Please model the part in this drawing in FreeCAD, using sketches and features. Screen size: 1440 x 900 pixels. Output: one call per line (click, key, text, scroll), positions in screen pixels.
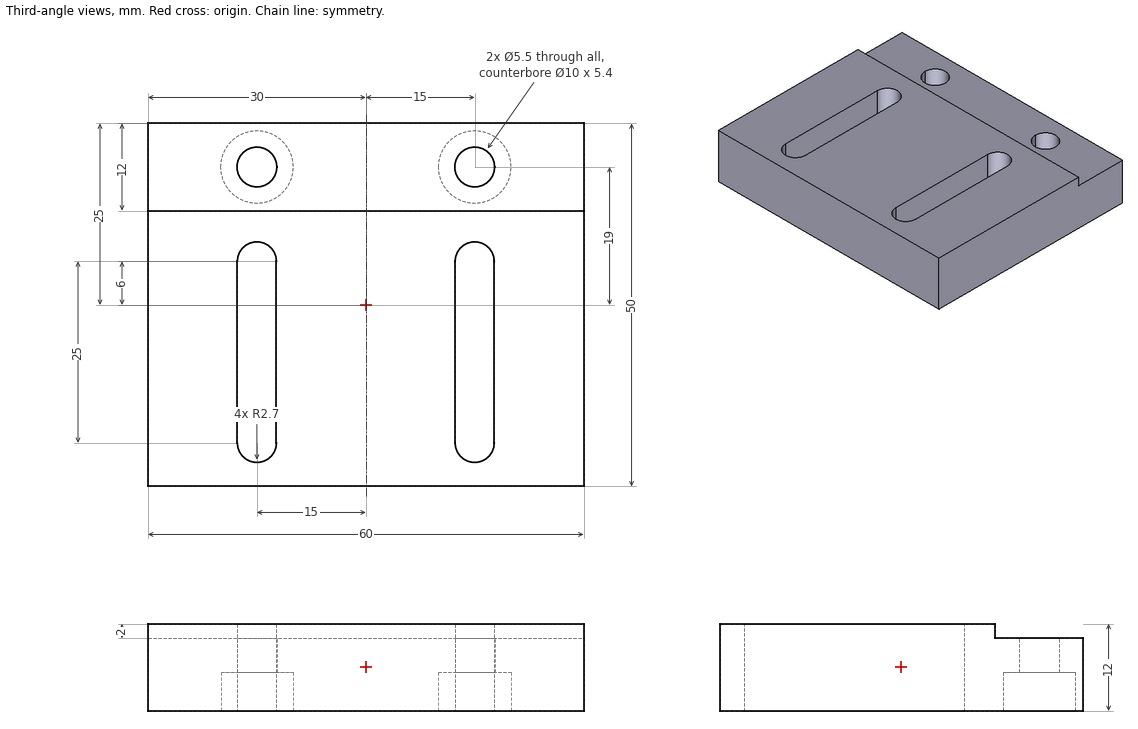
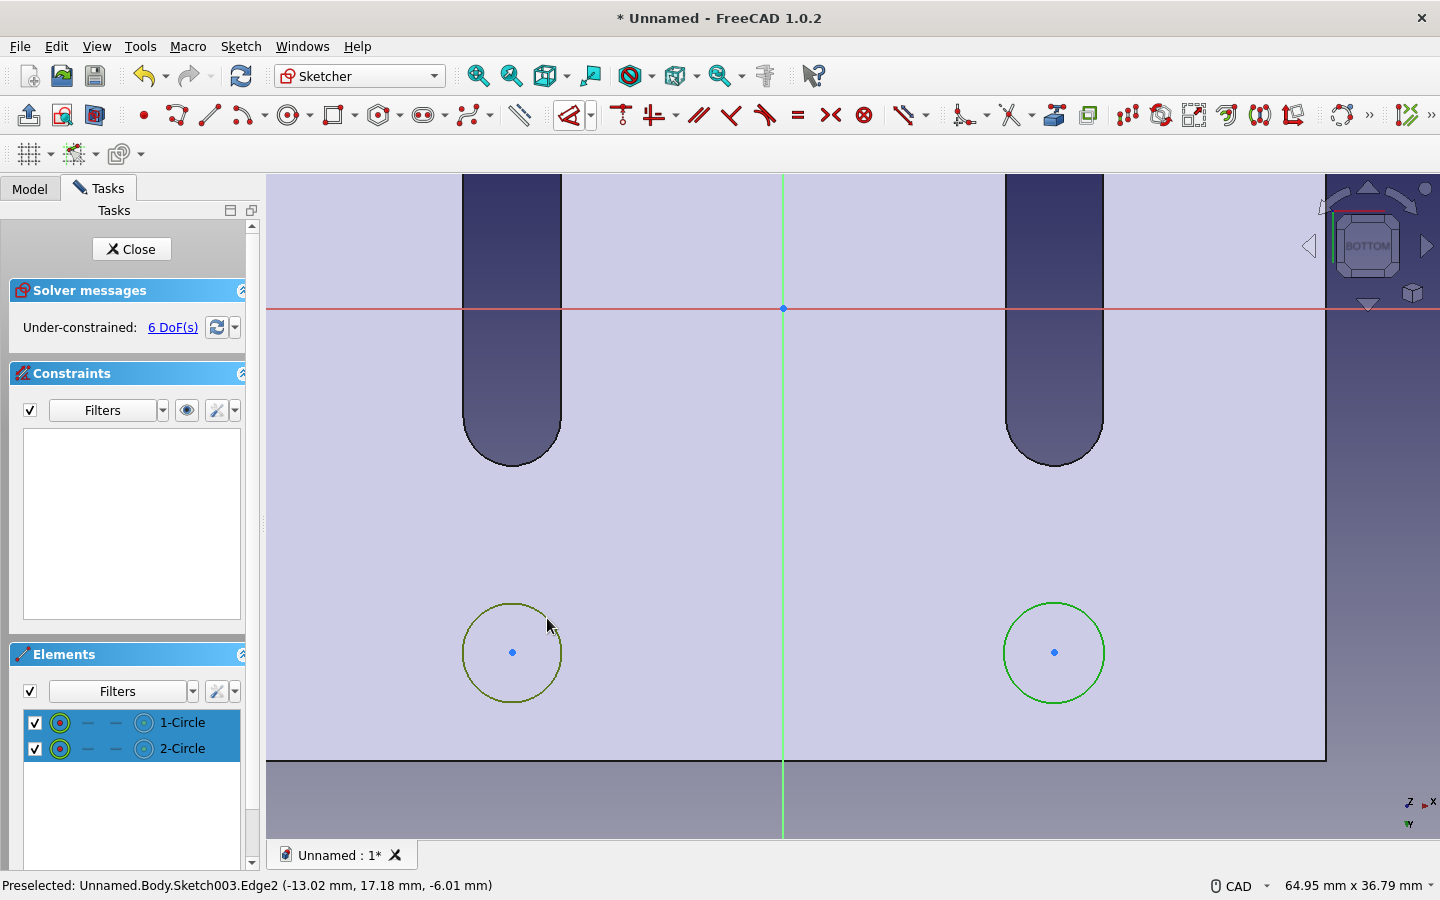
key(e)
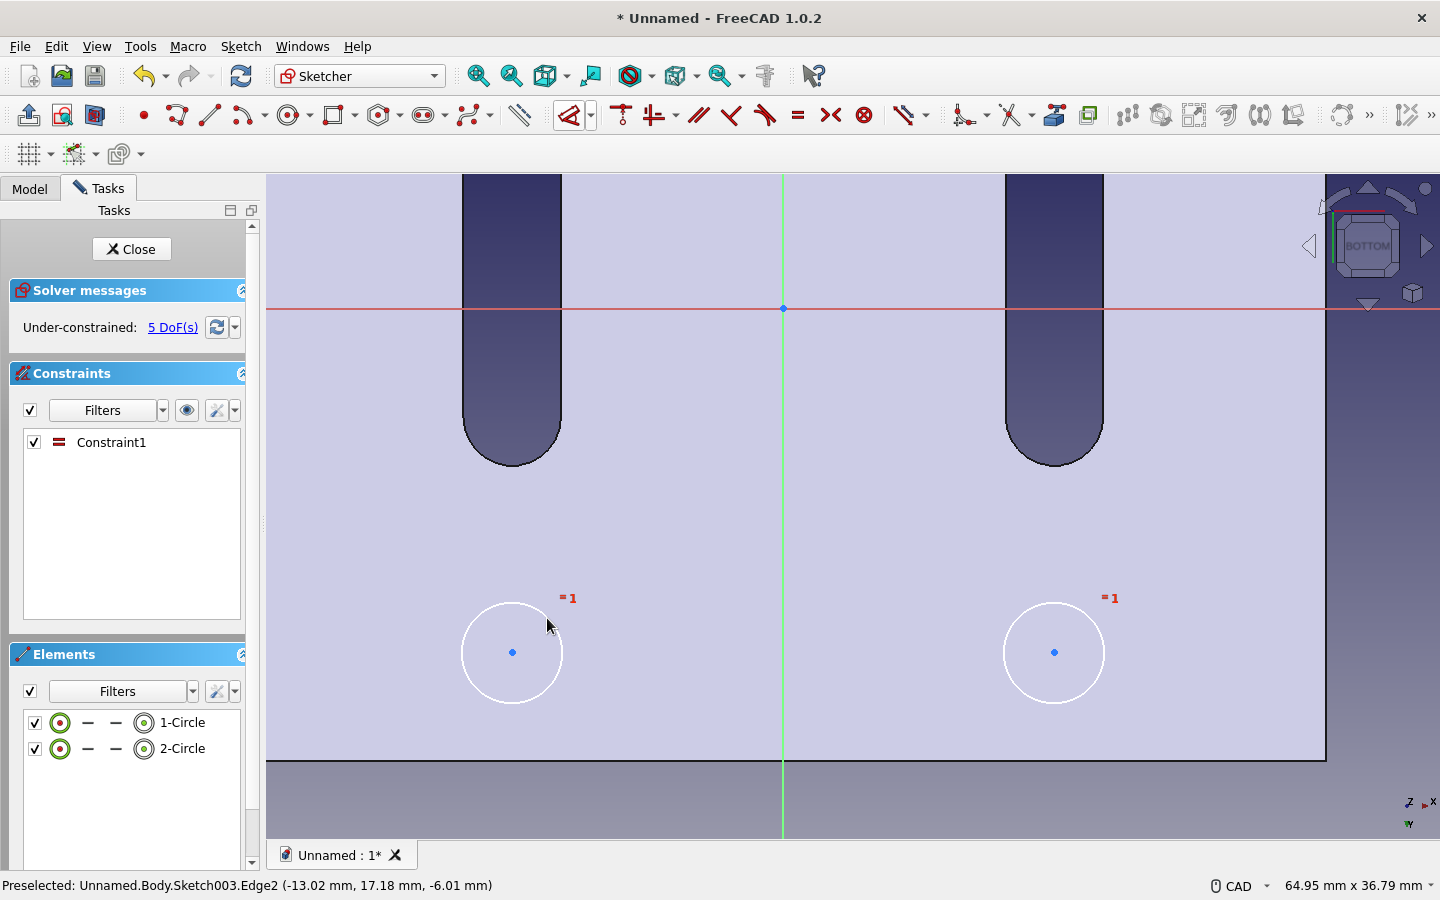
click(1054, 653)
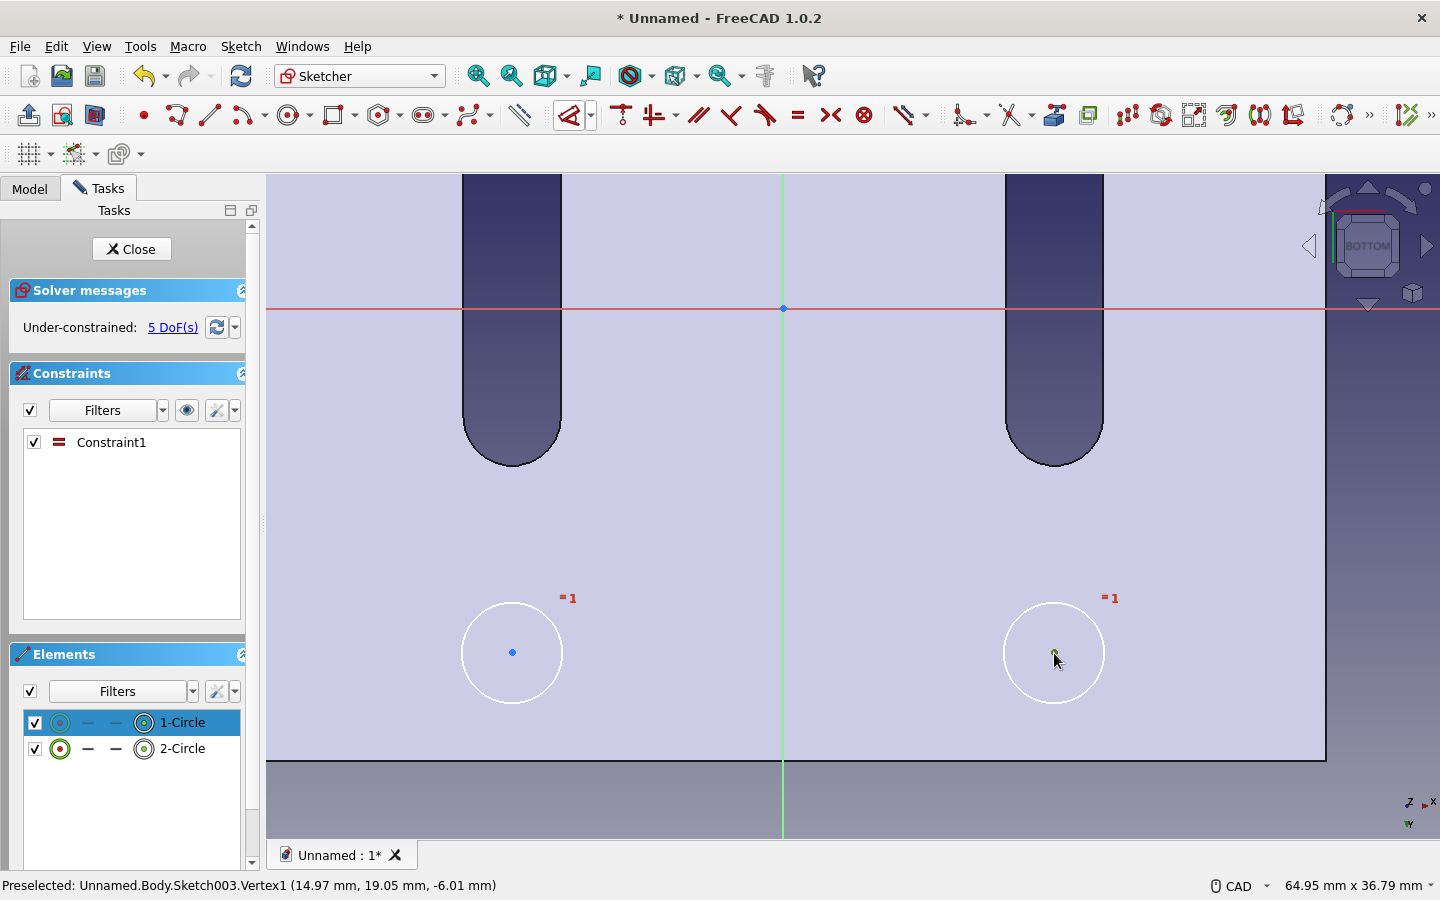
click(512, 653)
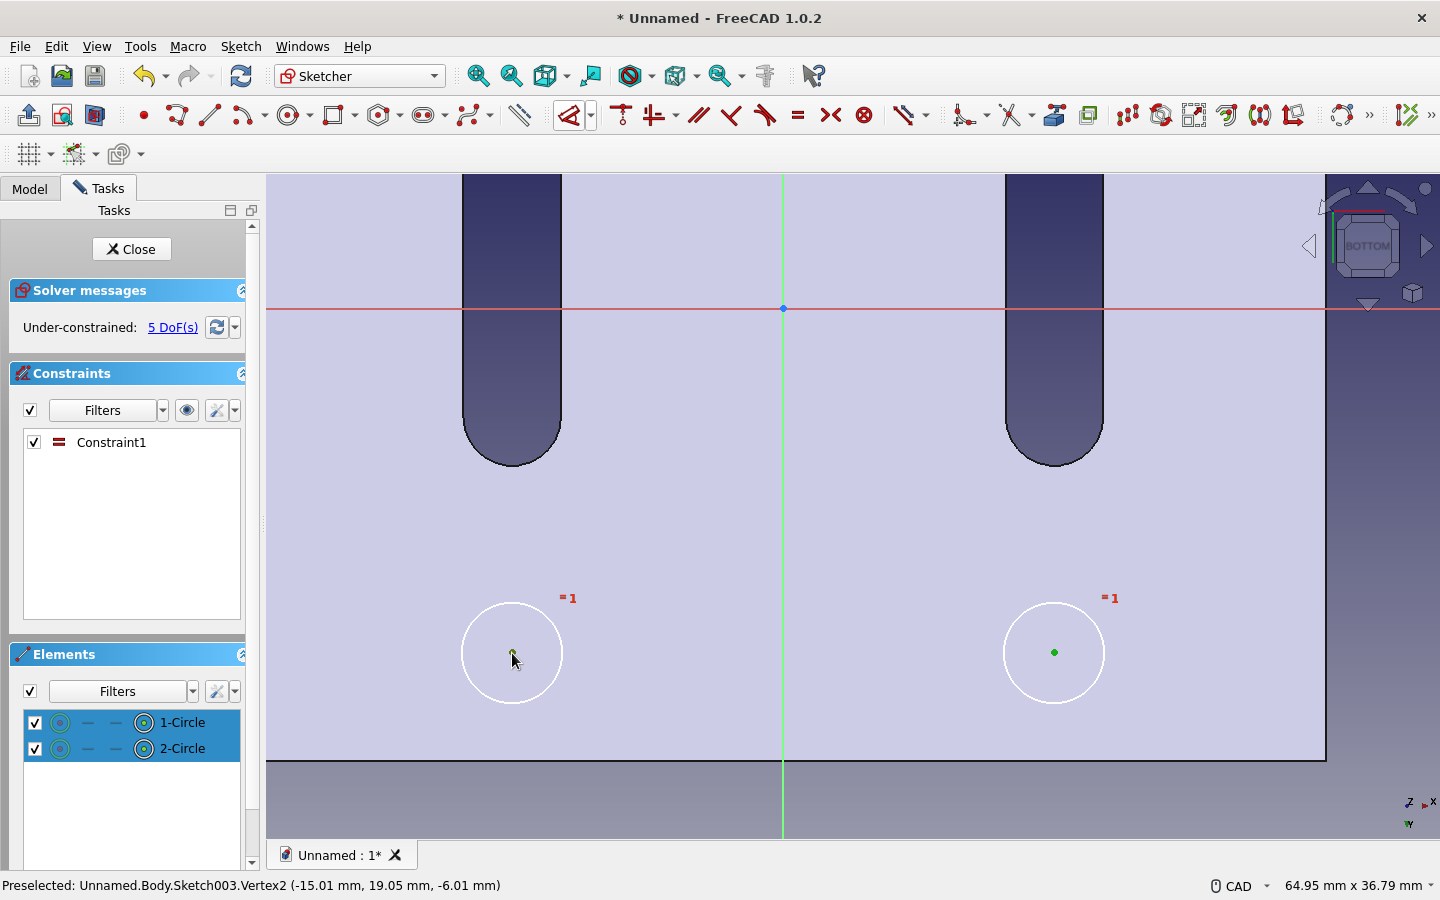
click(676, 116)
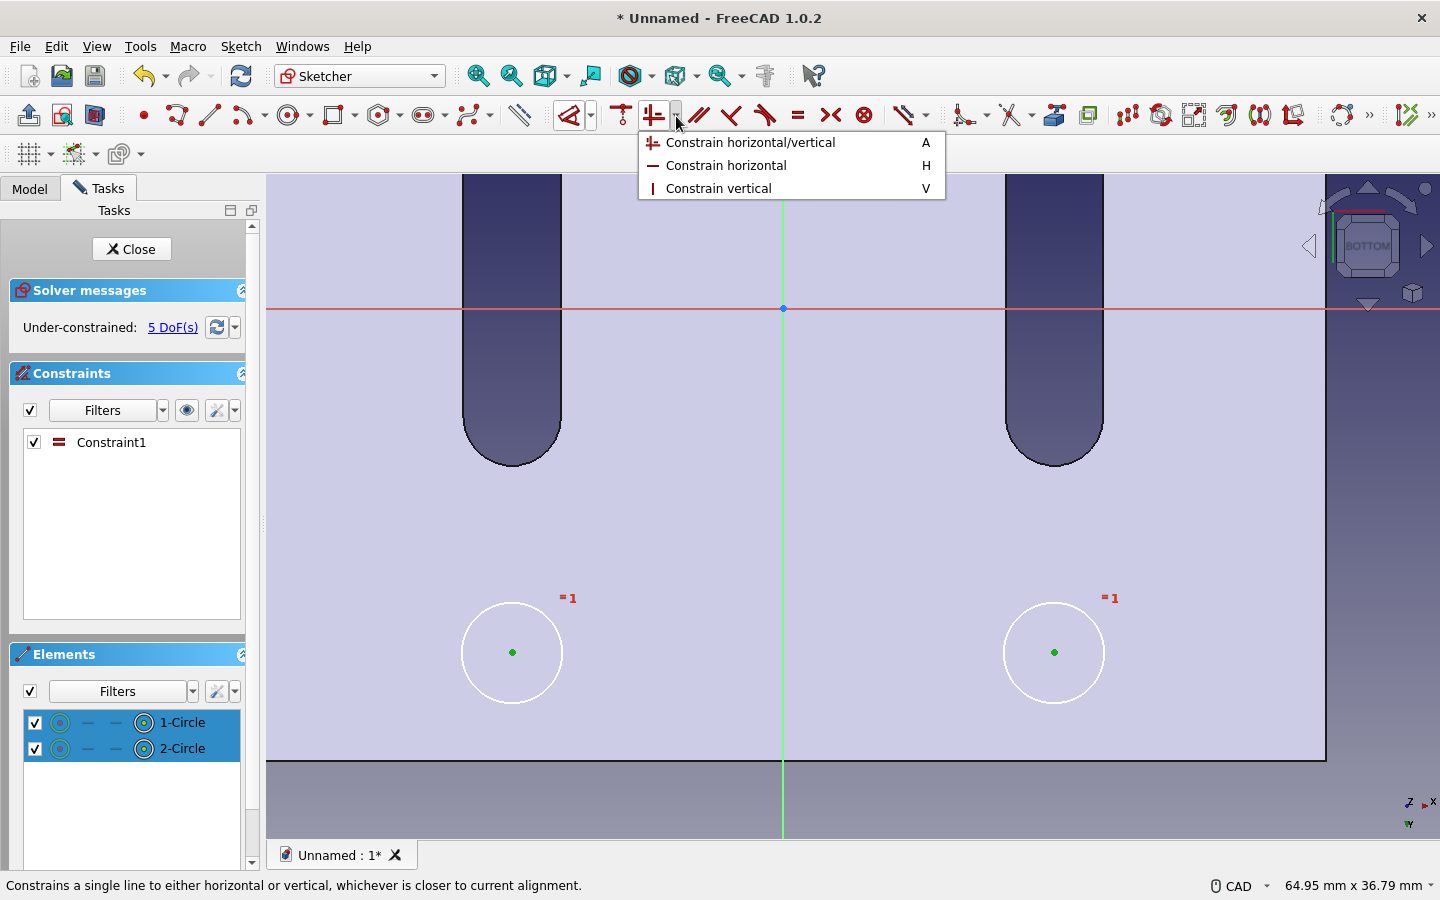
click(792, 166)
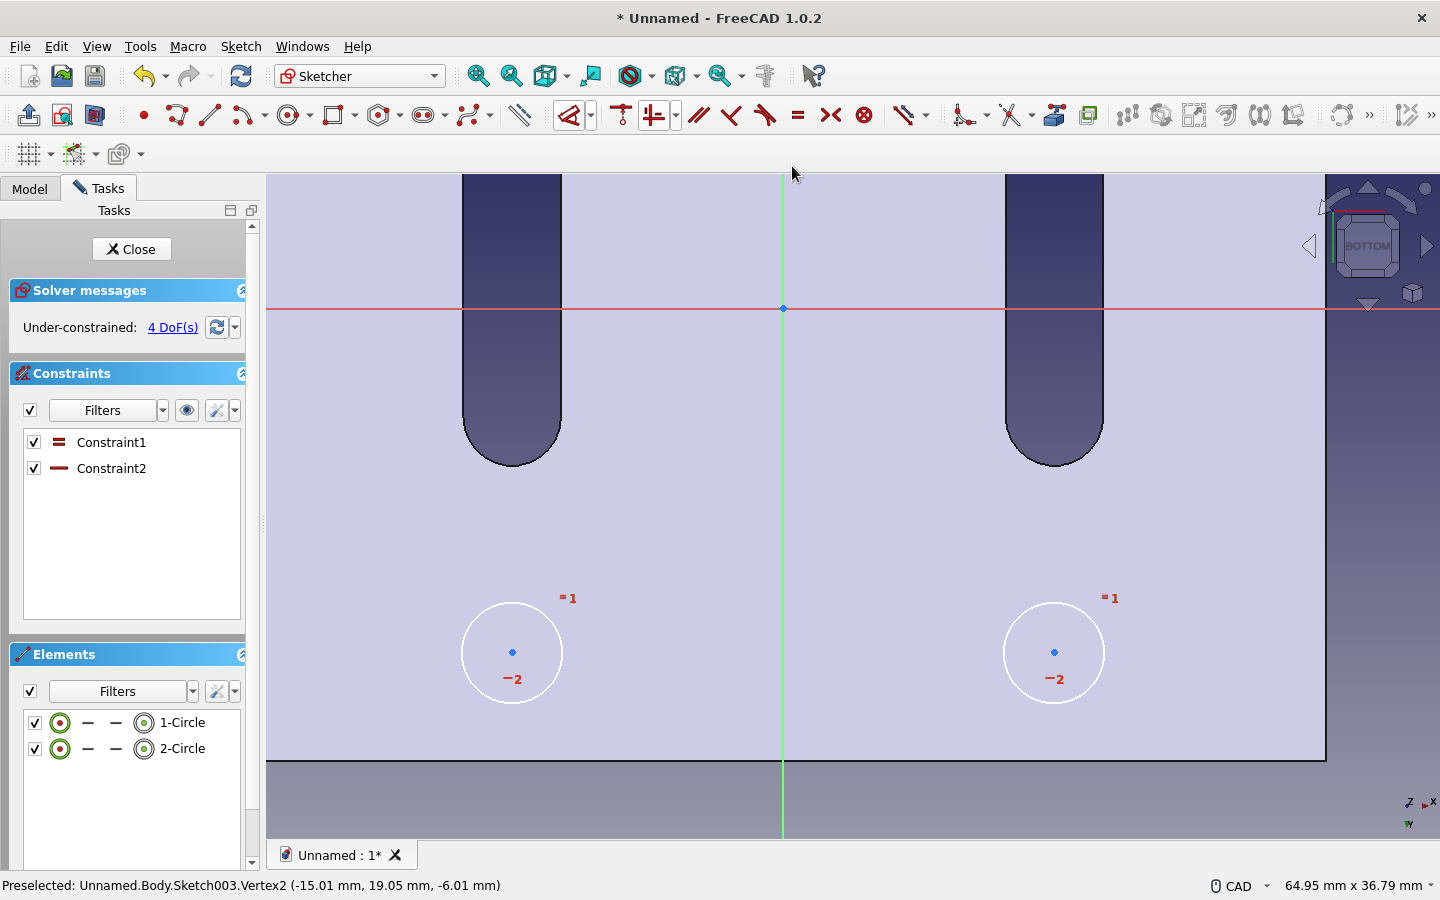
click(1089, 617)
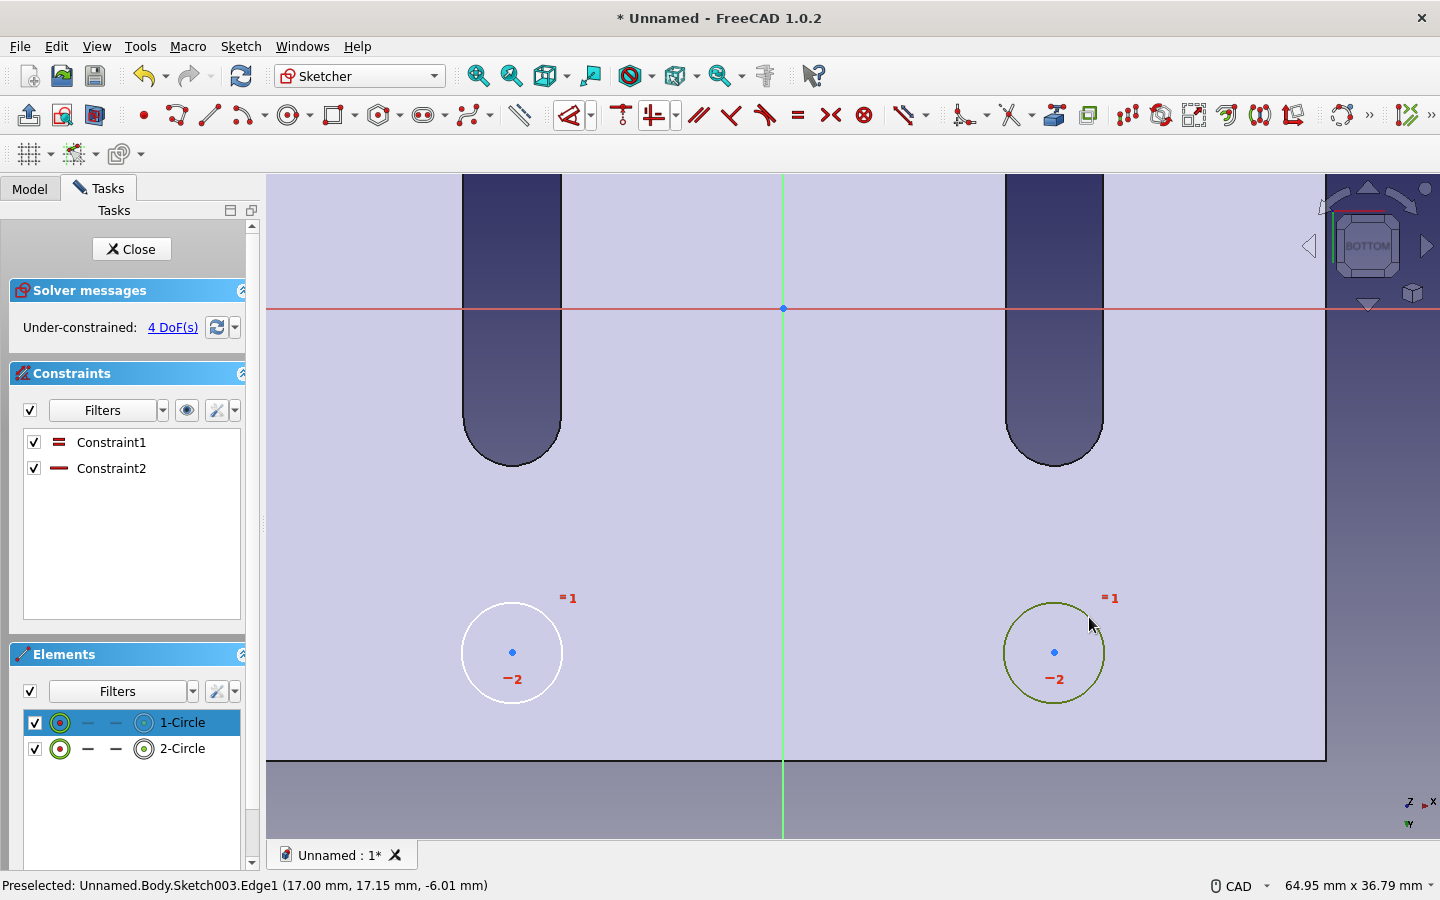
key(k)
key(o)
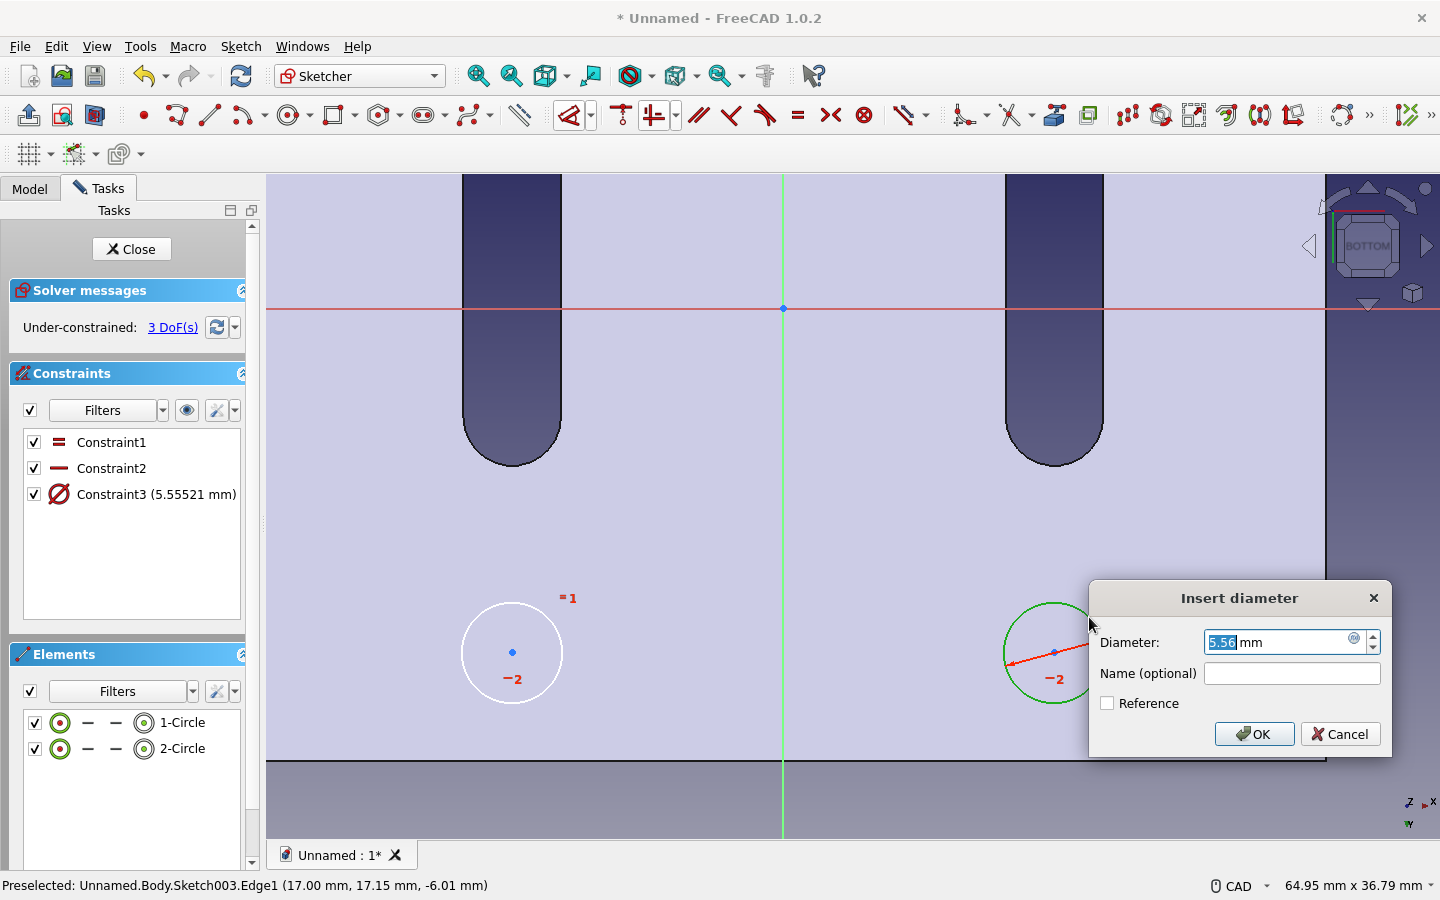
text(5.5)
key(Return)